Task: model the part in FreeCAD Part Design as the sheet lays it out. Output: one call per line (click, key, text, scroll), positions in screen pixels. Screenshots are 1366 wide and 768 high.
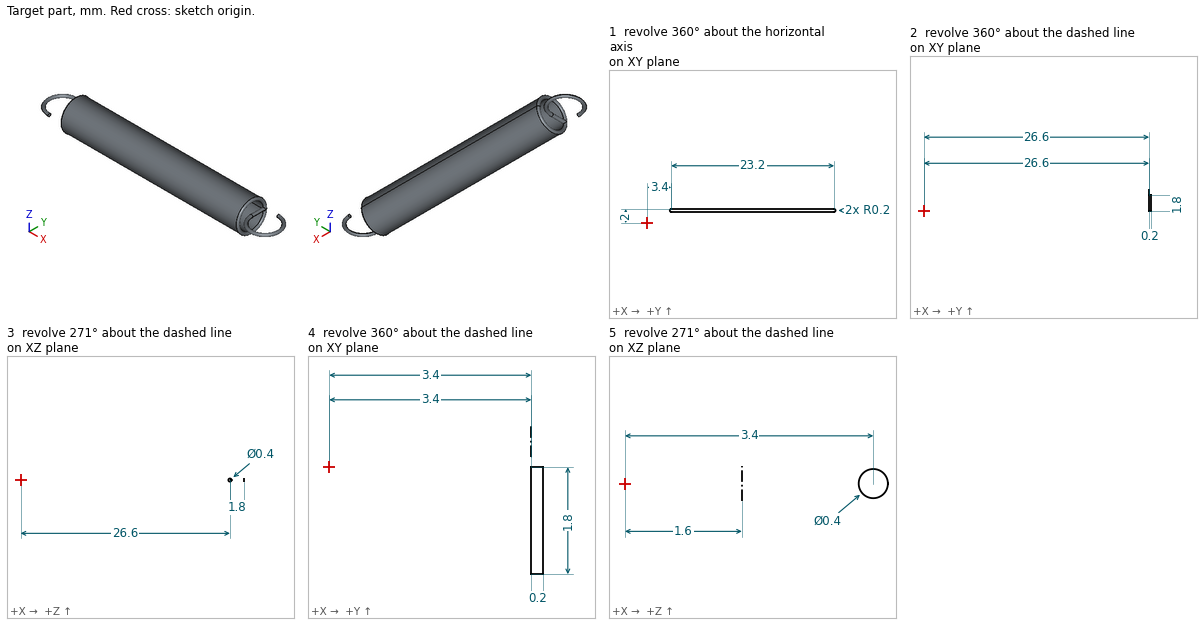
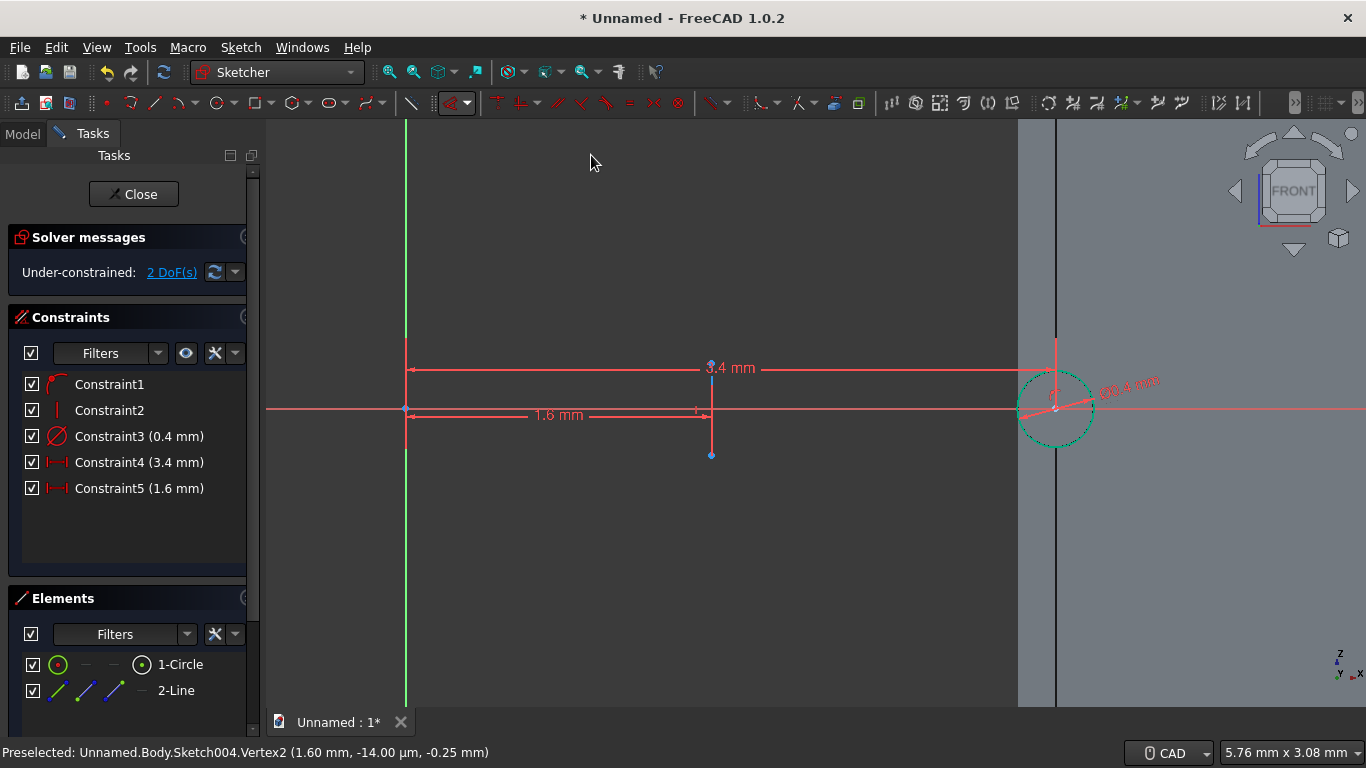
click(134, 194)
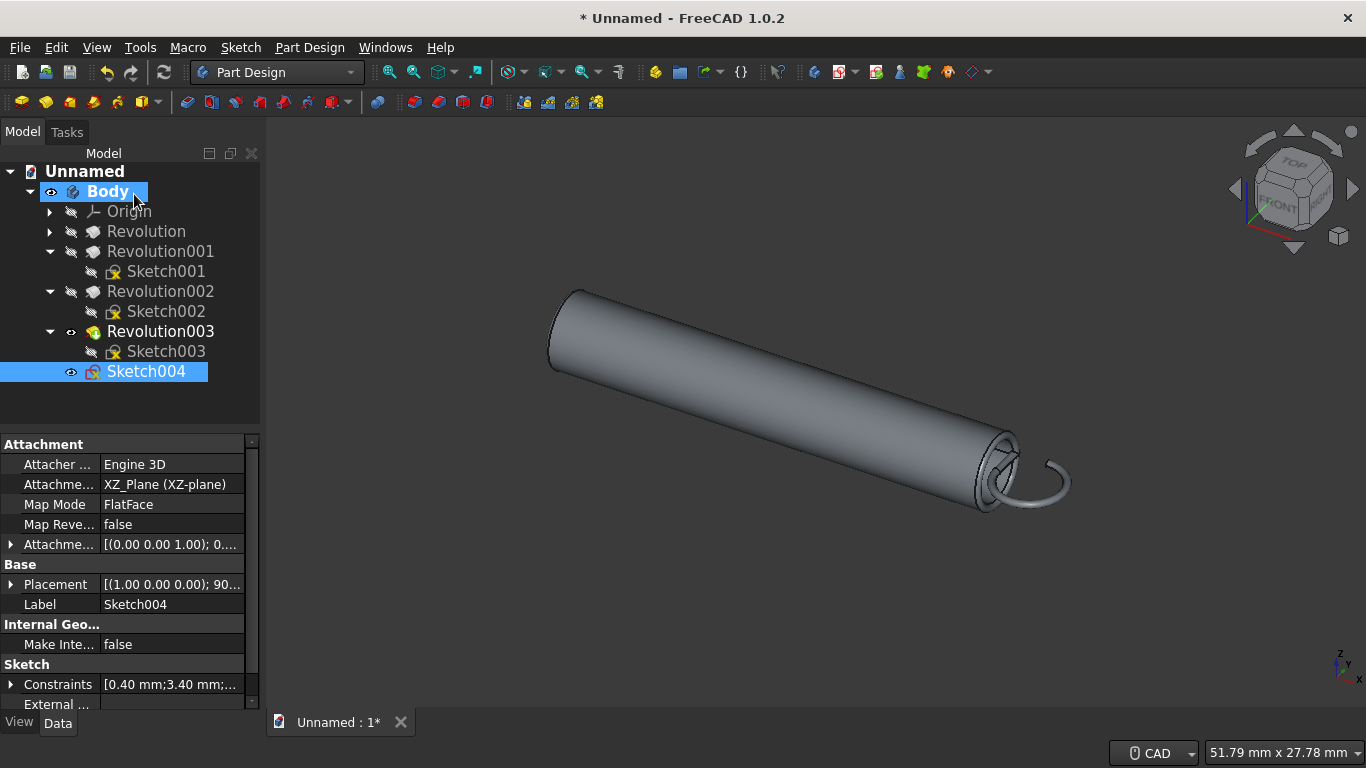
click(46, 102)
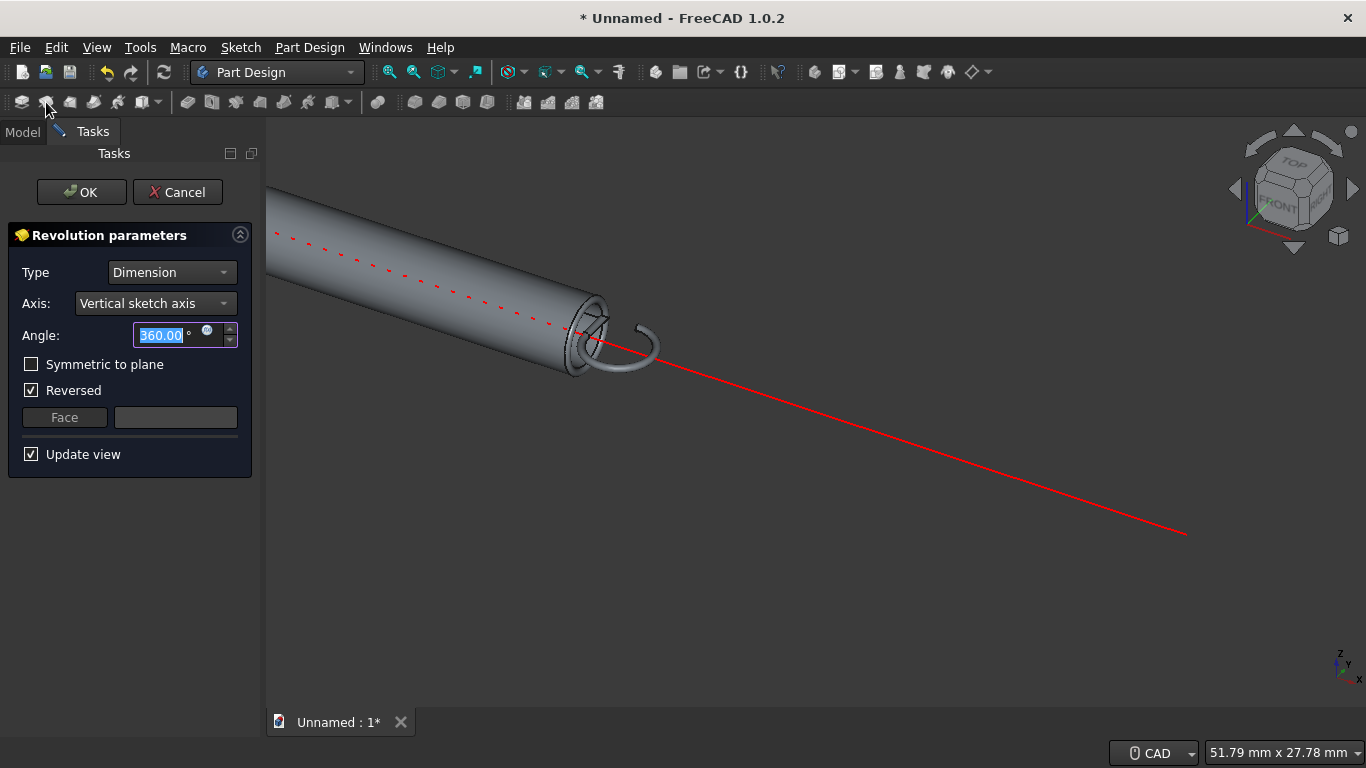
click(156, 304)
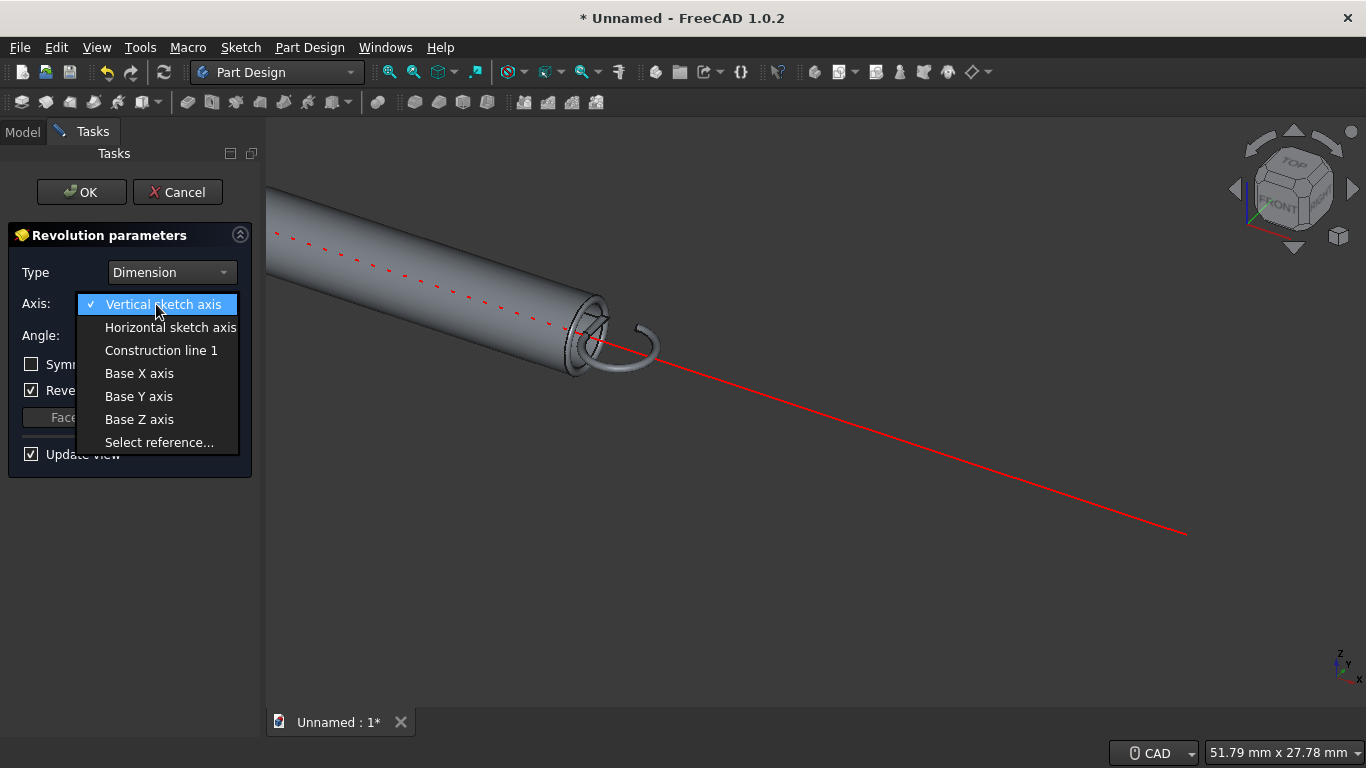
click(156, 350)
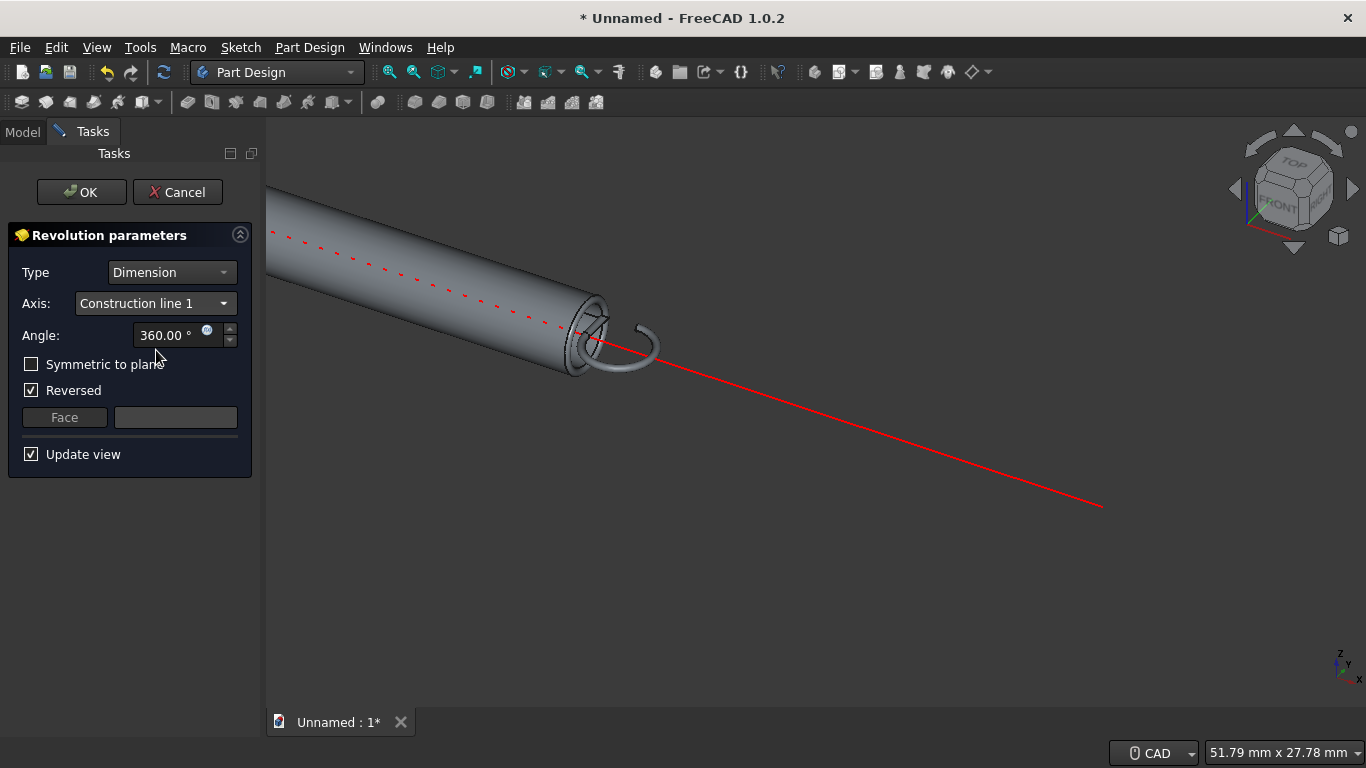
triple_click(178, 335)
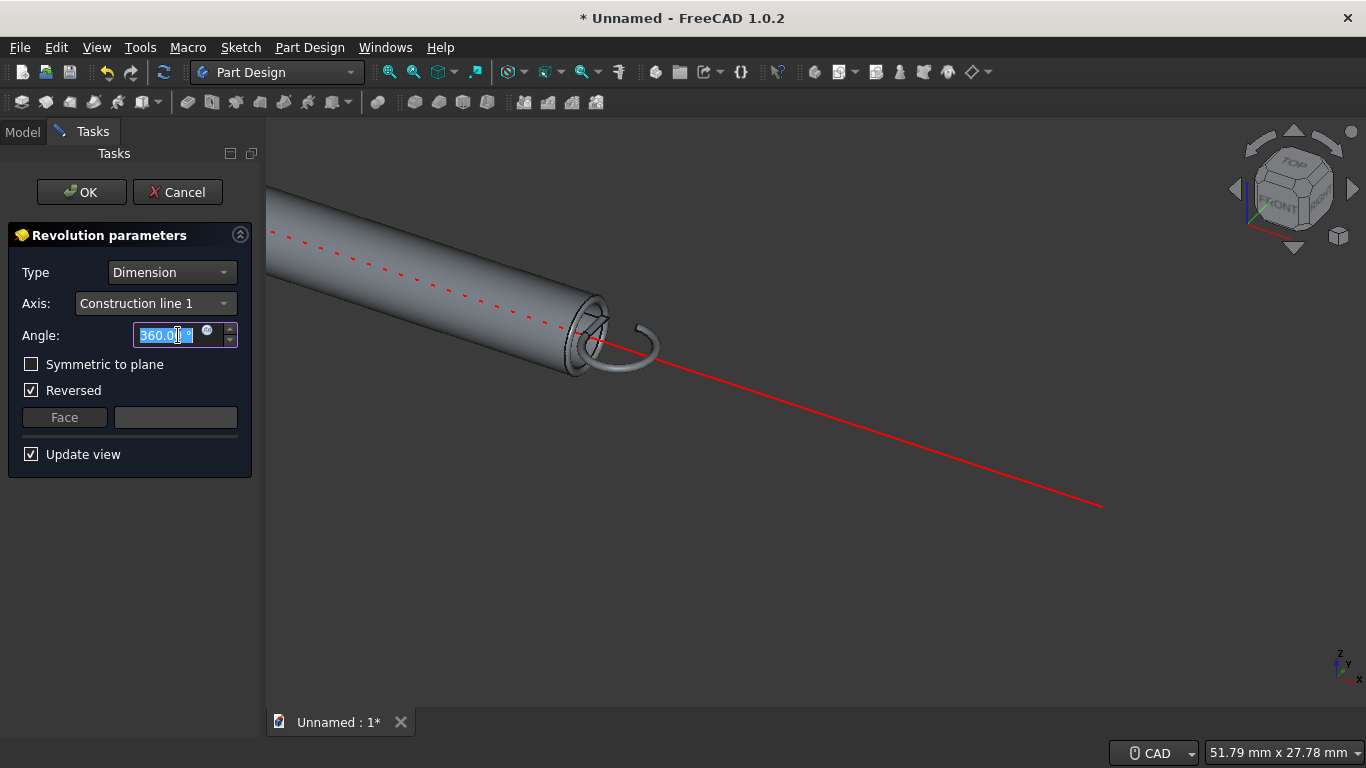
text(271)
key(Tab)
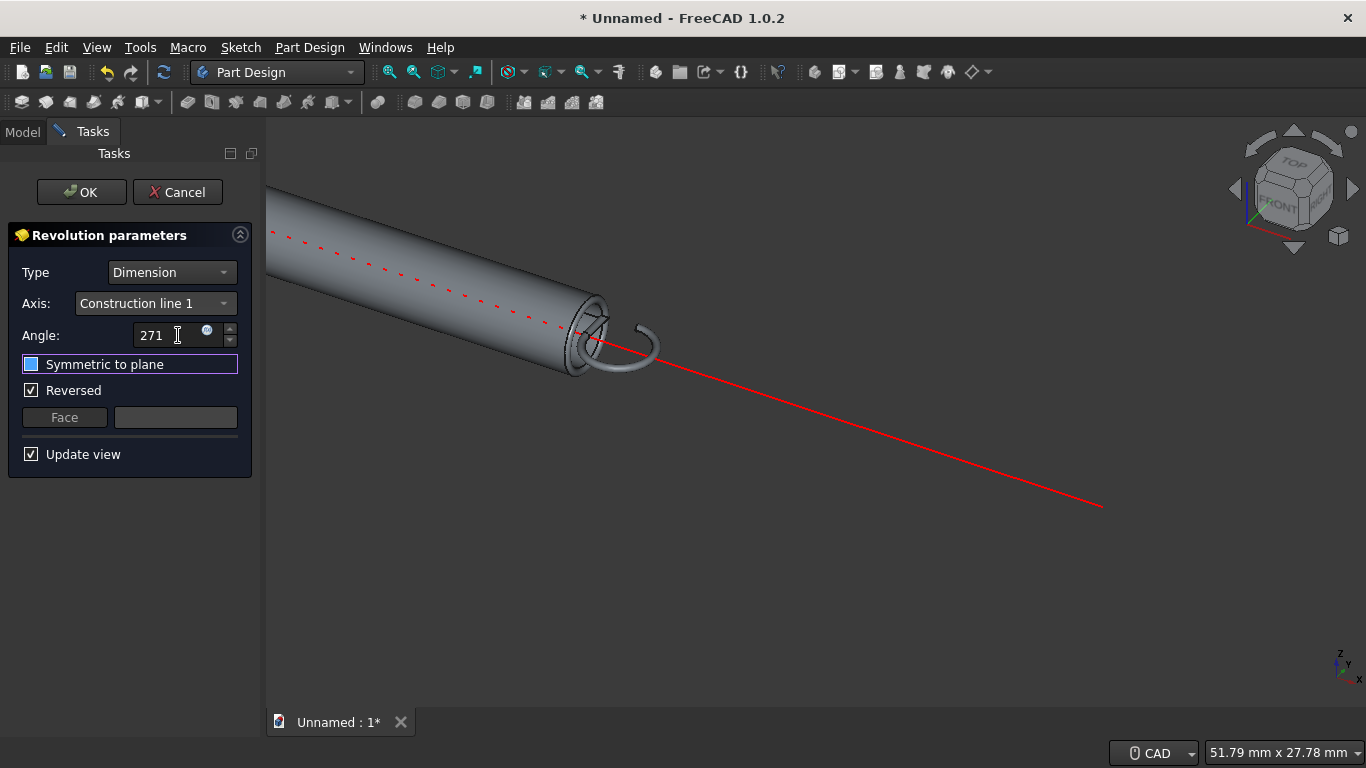
click(30, 390)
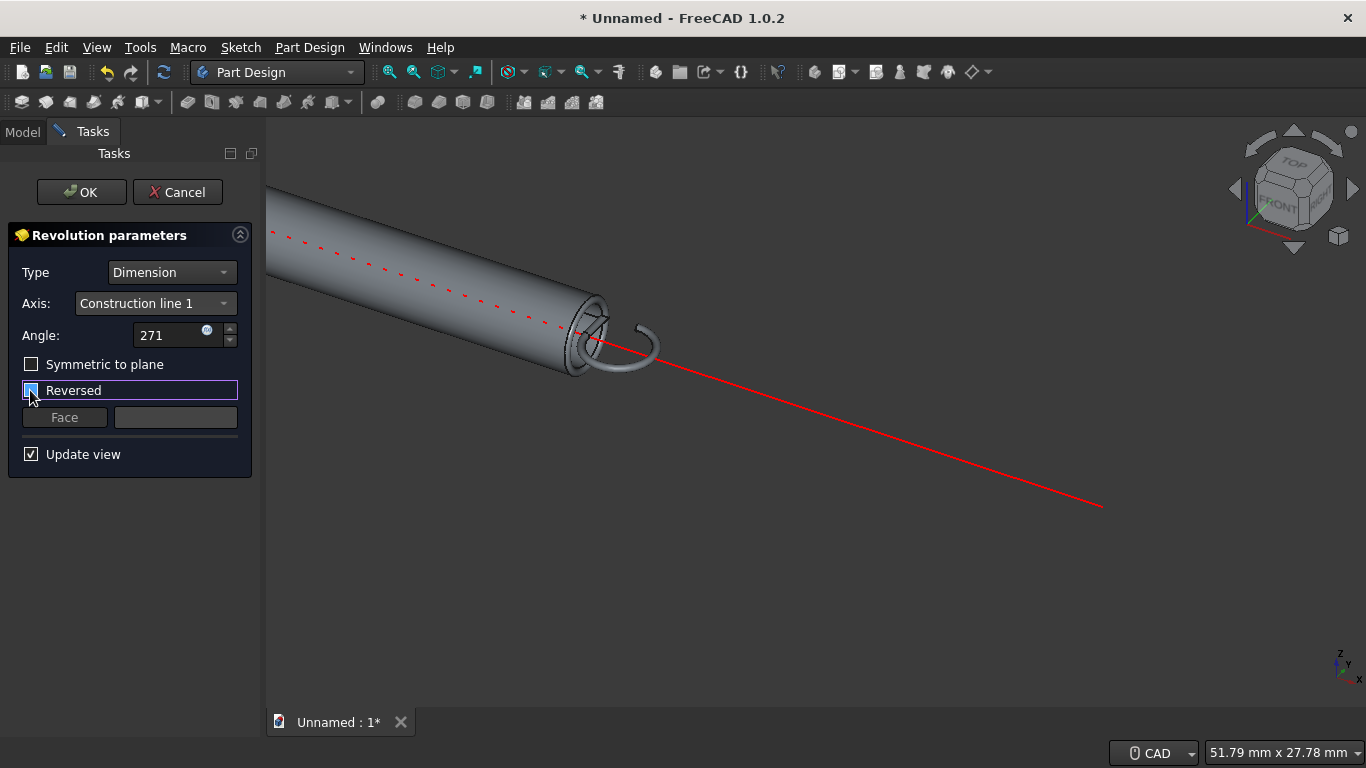
click(82, 192)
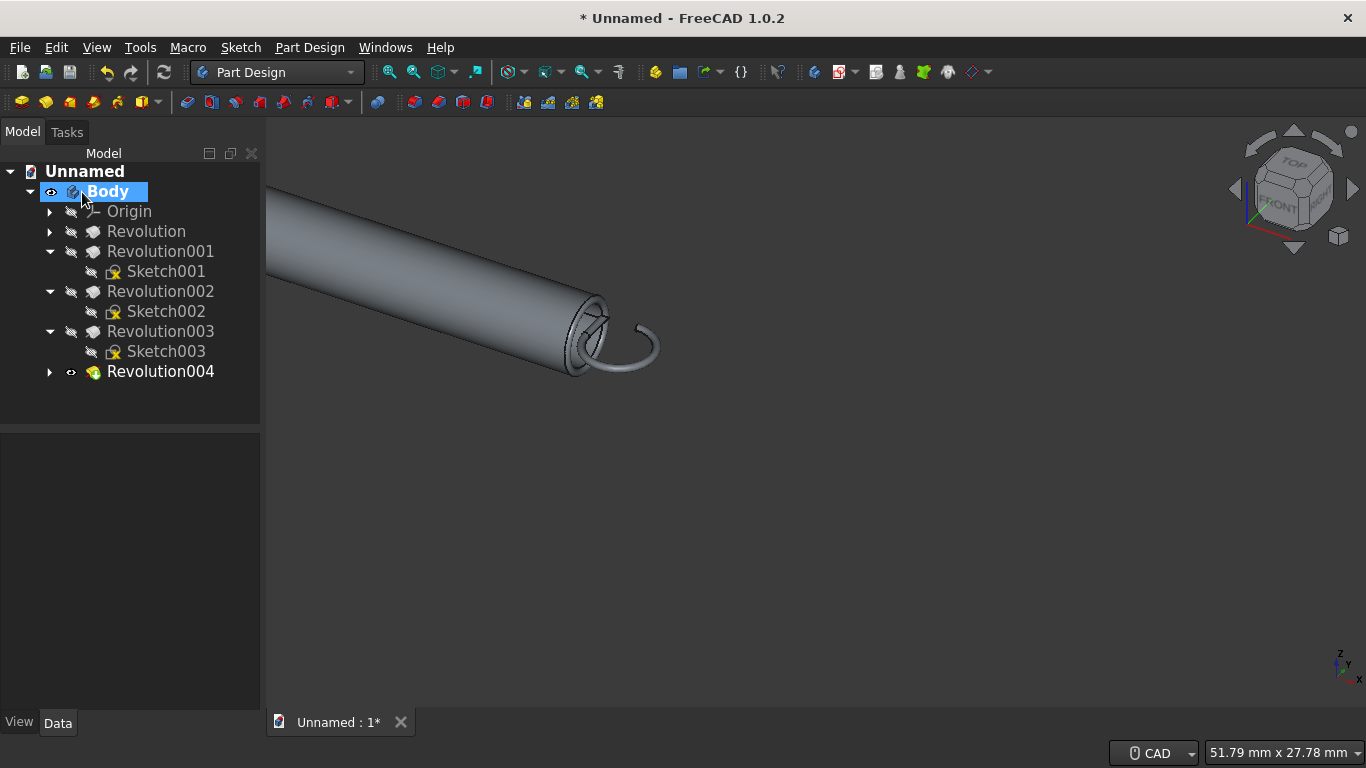
key(0)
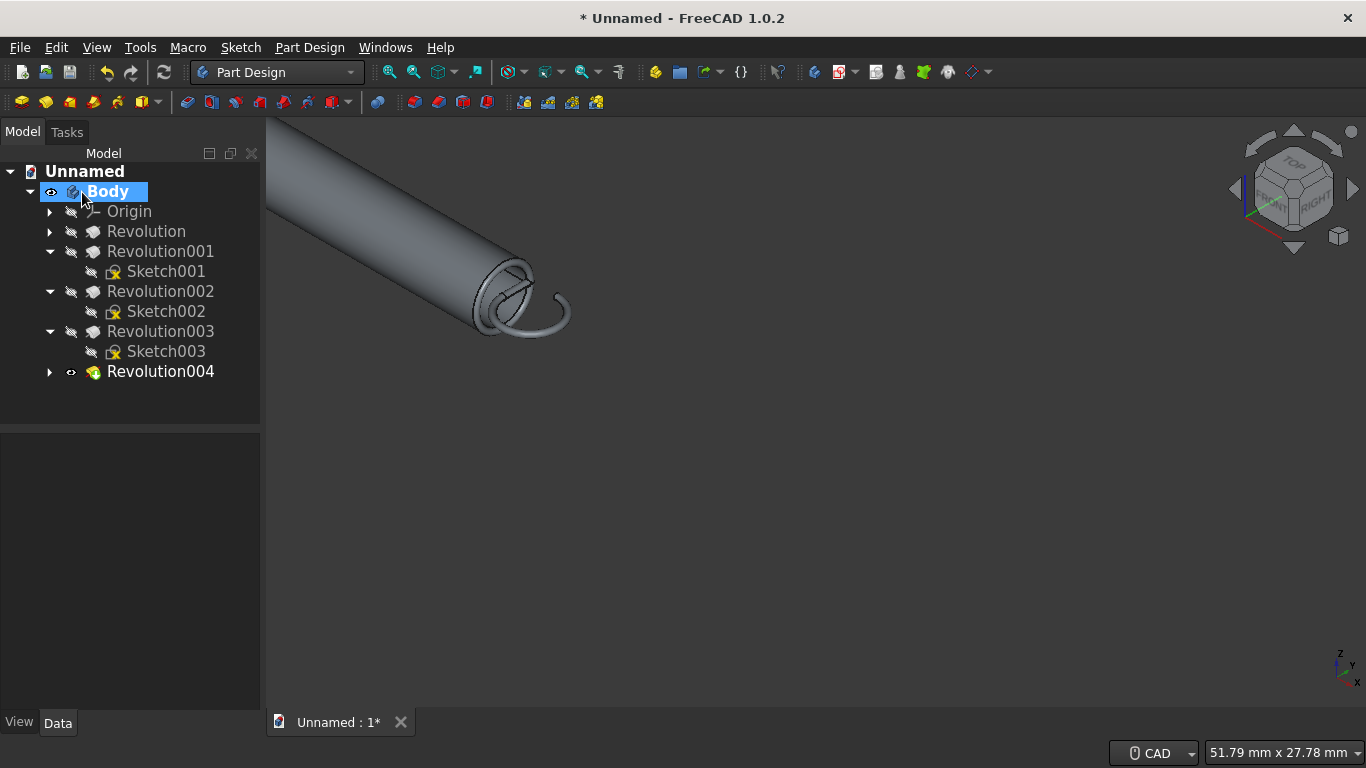
key(v)
key(f)